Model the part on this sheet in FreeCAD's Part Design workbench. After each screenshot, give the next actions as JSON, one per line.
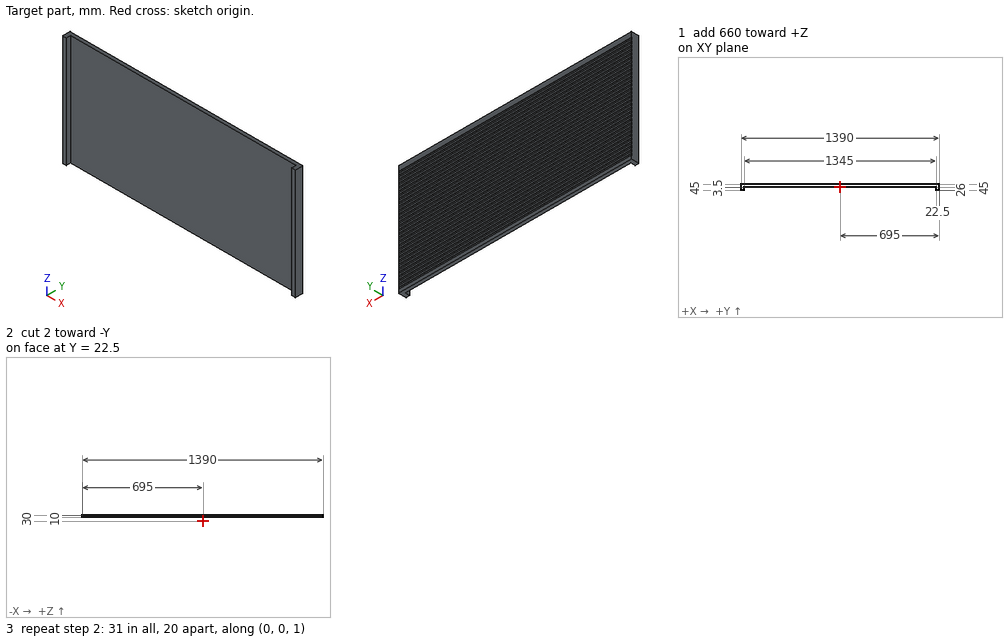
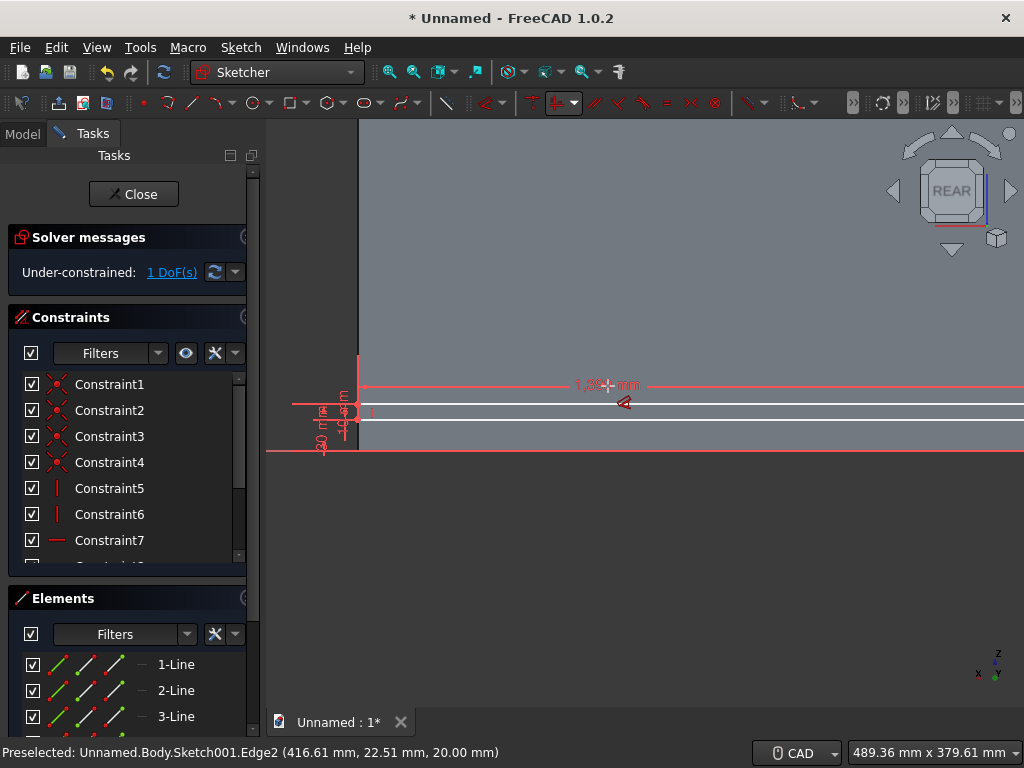
{"action": "left_click", "coordinate": [358, 404]}
{"action": "left_click", "coordinate": [608, 485]}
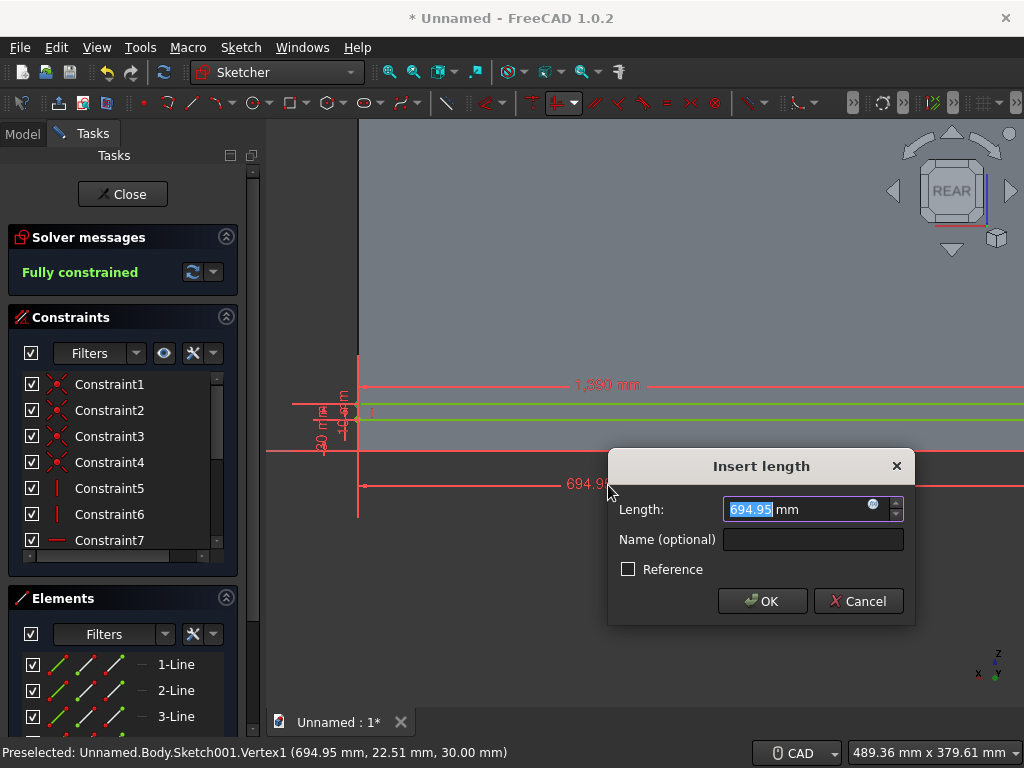
{"action": "type", "text": "695"}
{"action": "key", "text": "Return"}
{"action": "key", "text": "Escape"}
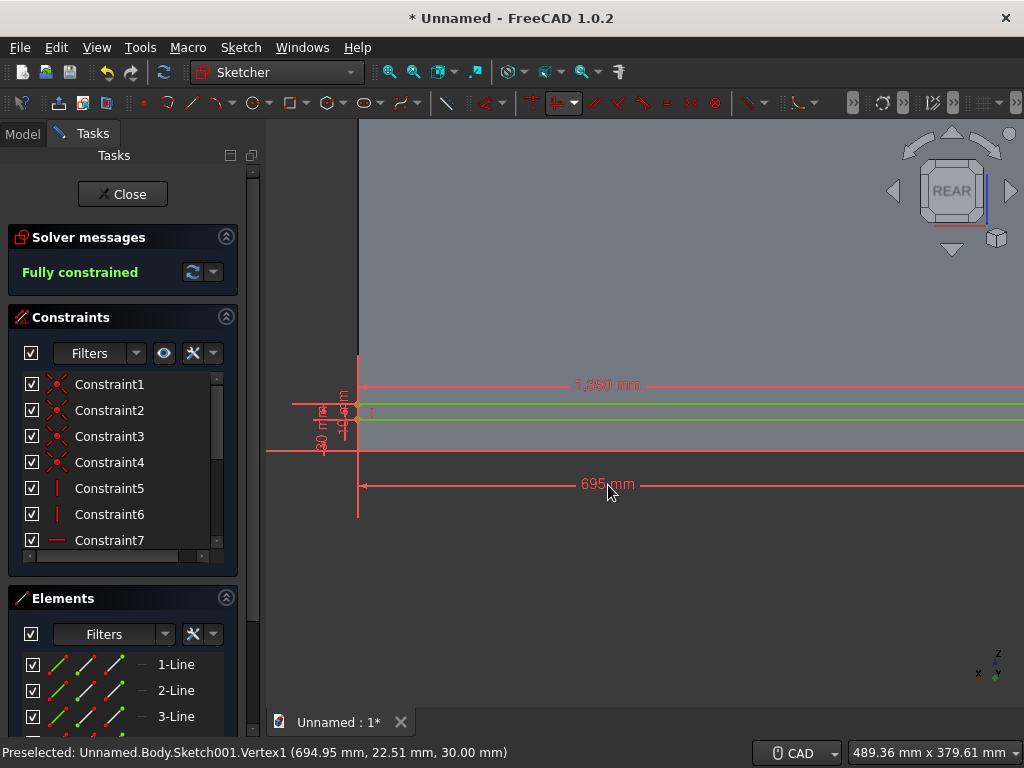
{"action": "left_click", "coordinate": [123, 194]}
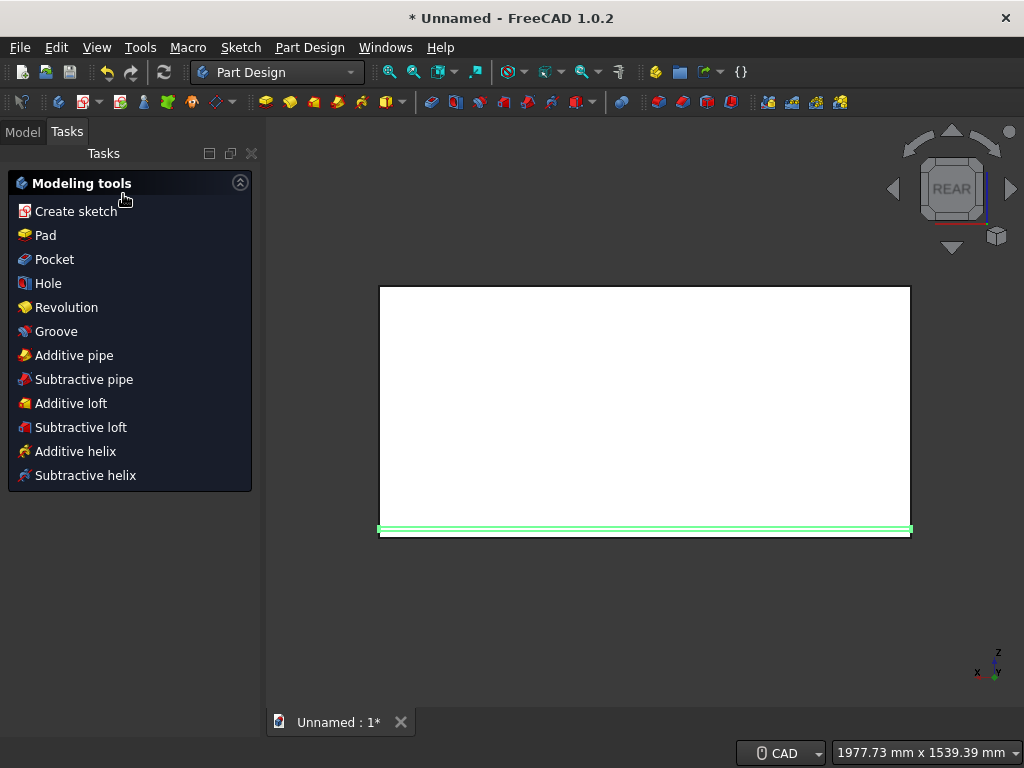
{"action": "left_click", "coordinate": [432, 102]}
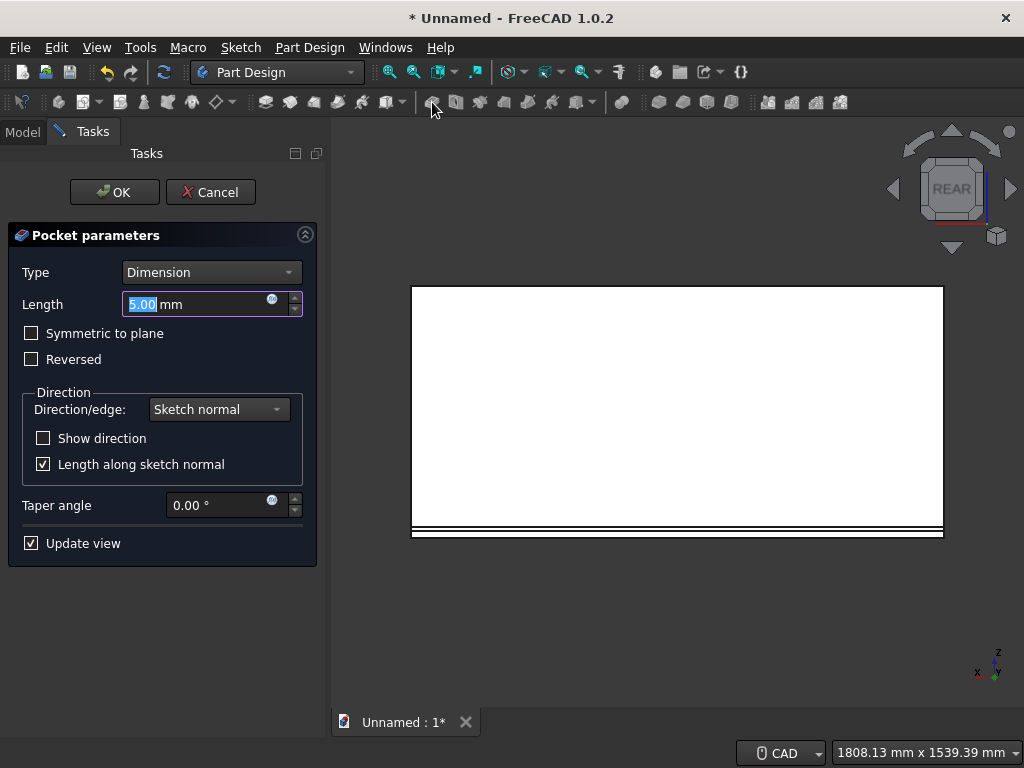
{"action": "type", "text": "2"}
{"action": "key", "text": "Tab"}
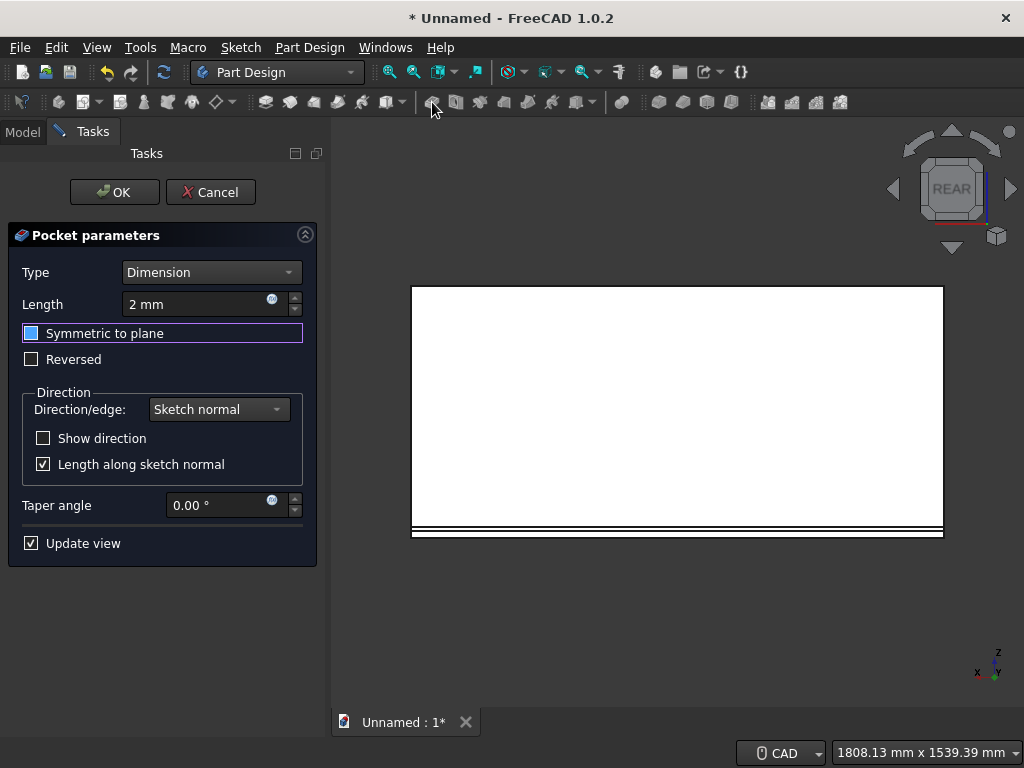
{"action": "left_click", "coordinate": [115, 192]}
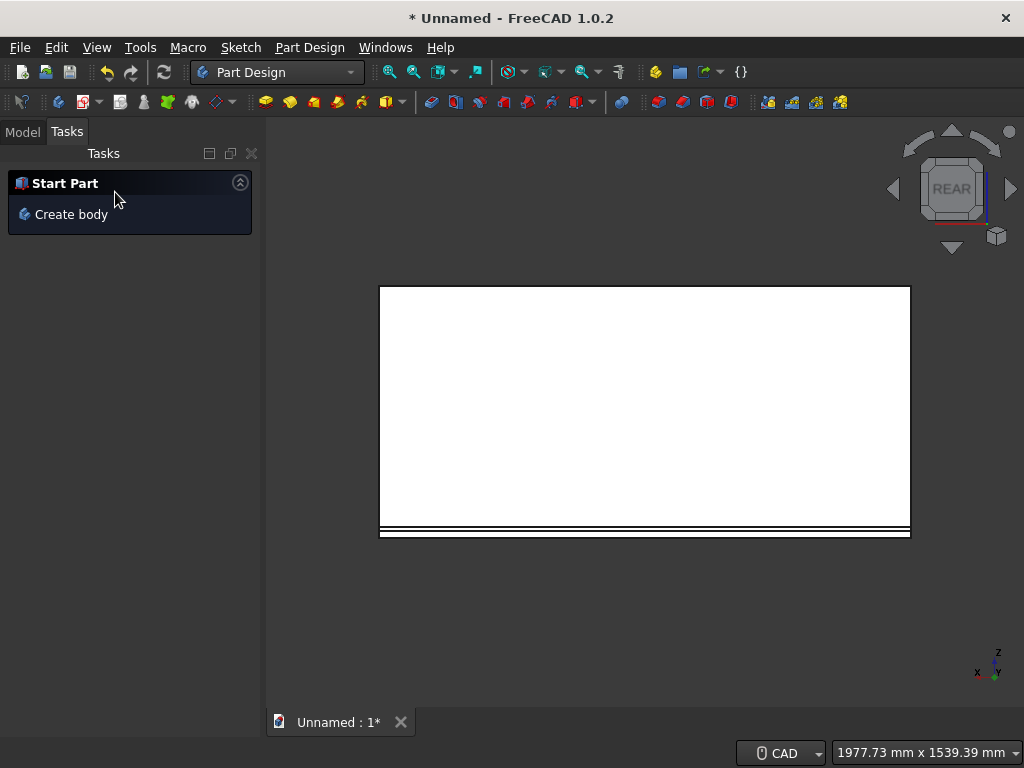
{"action": "left_click", "coordinate": [23, 131]}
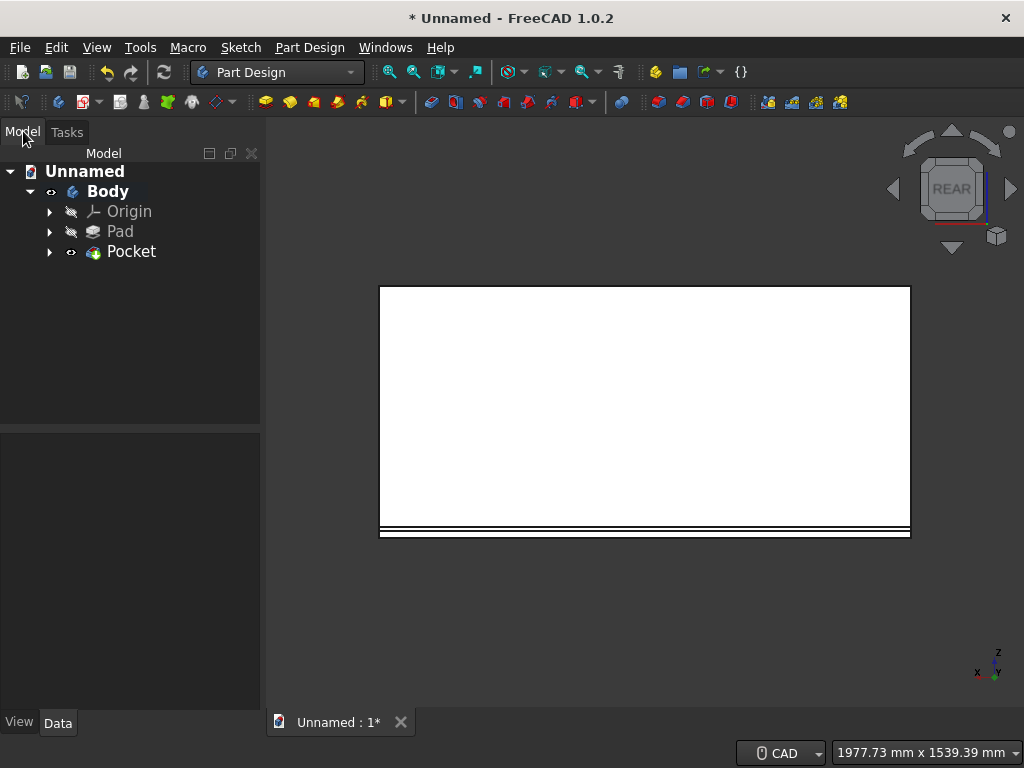
{"action": "left_click", "coordinate": [116, 252]}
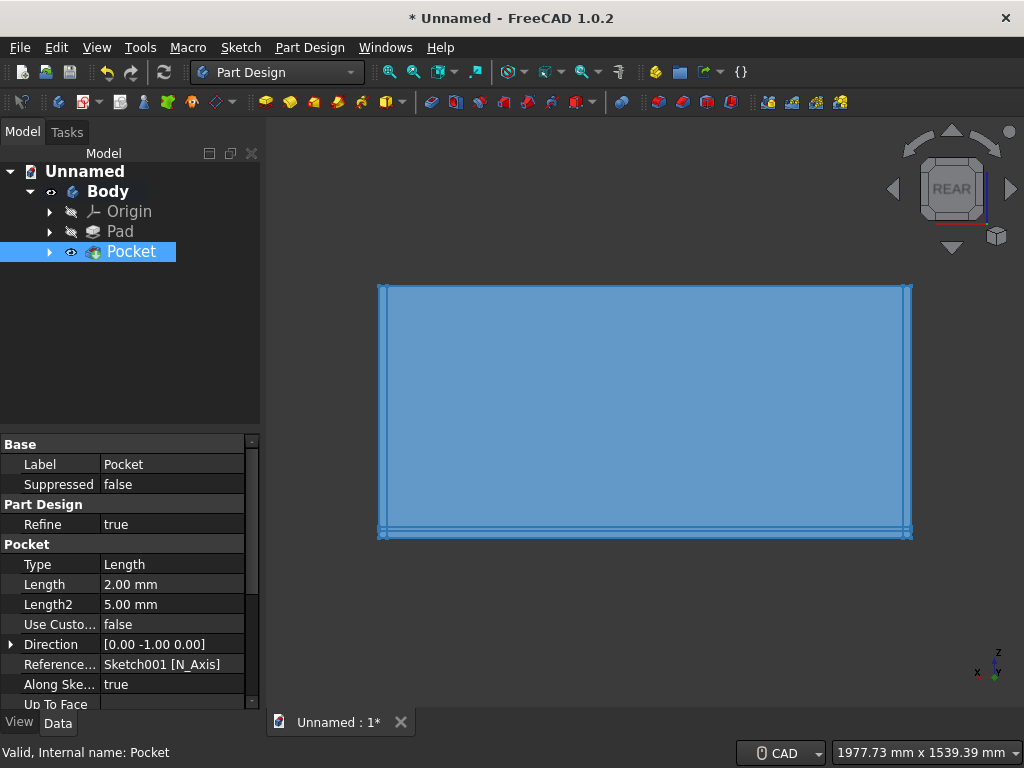
{"action": "left_click", "coordinate": [792, 102]}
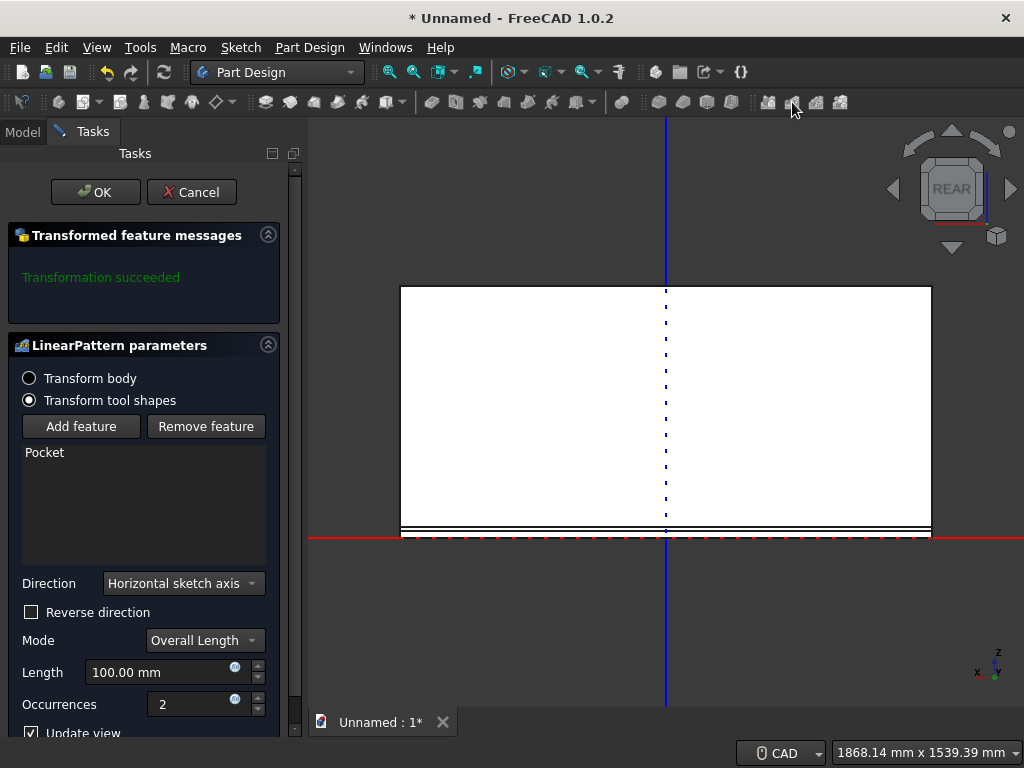
{"action": "left_click", "coordinate": [184, 584]}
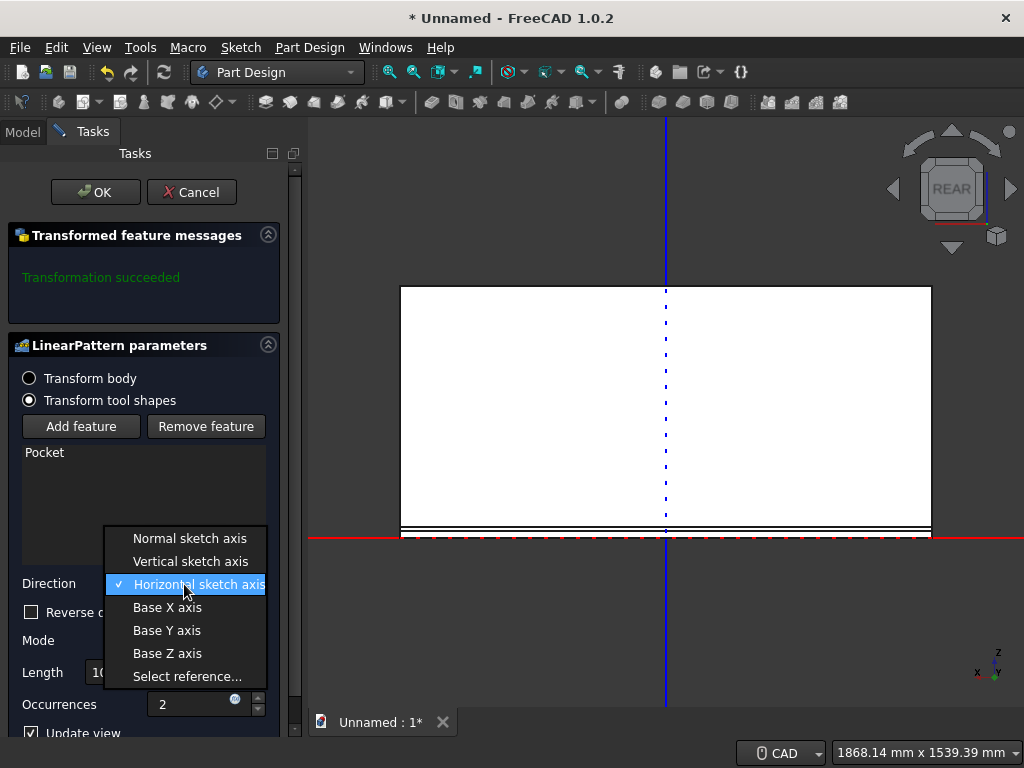
{"action": "left_click", "coordinate": [184, 654]}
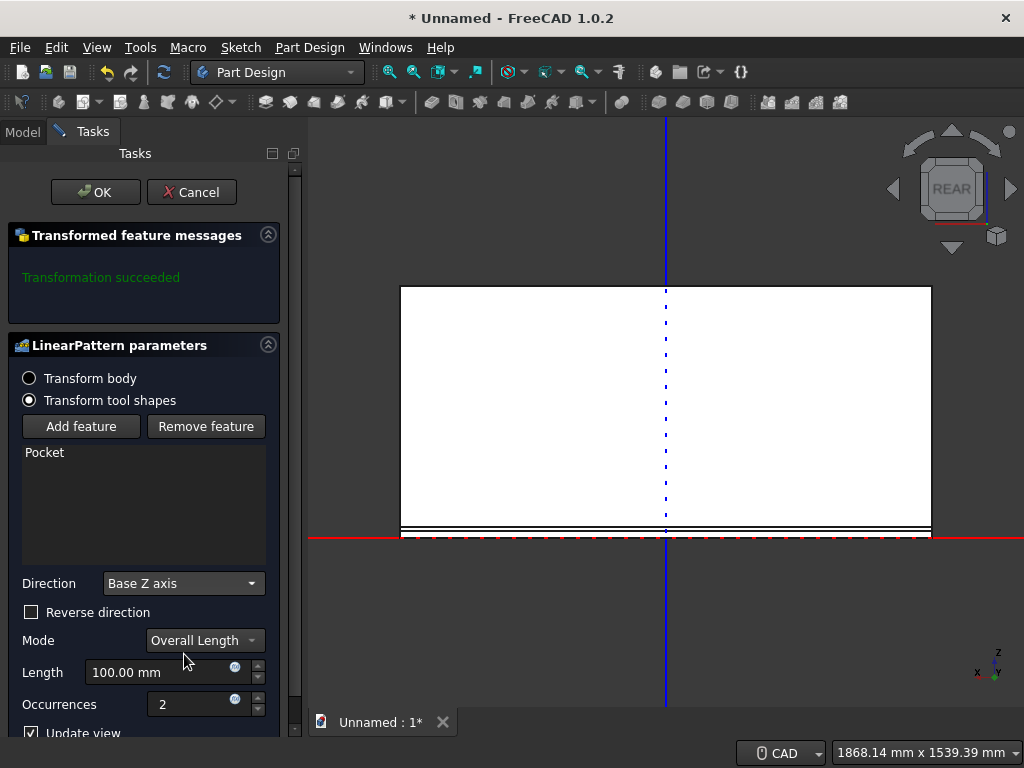
{"action": "left_click", "coordinate": [206, 640]}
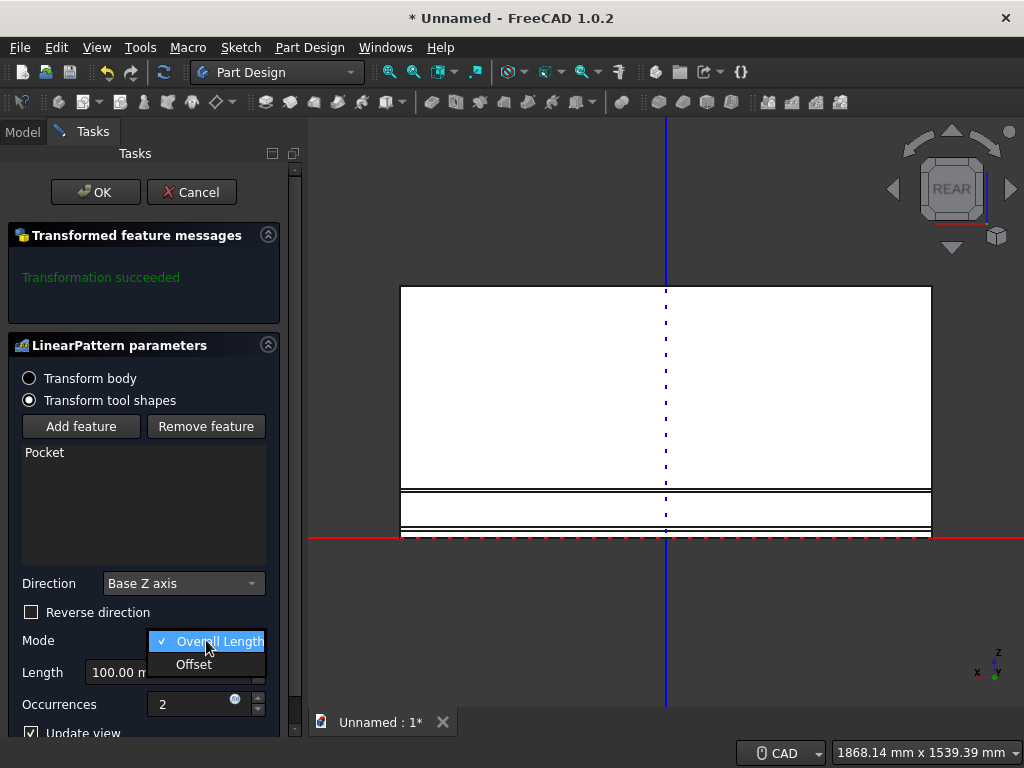
{"action": "left_click", "coordinate": [206, 664]}